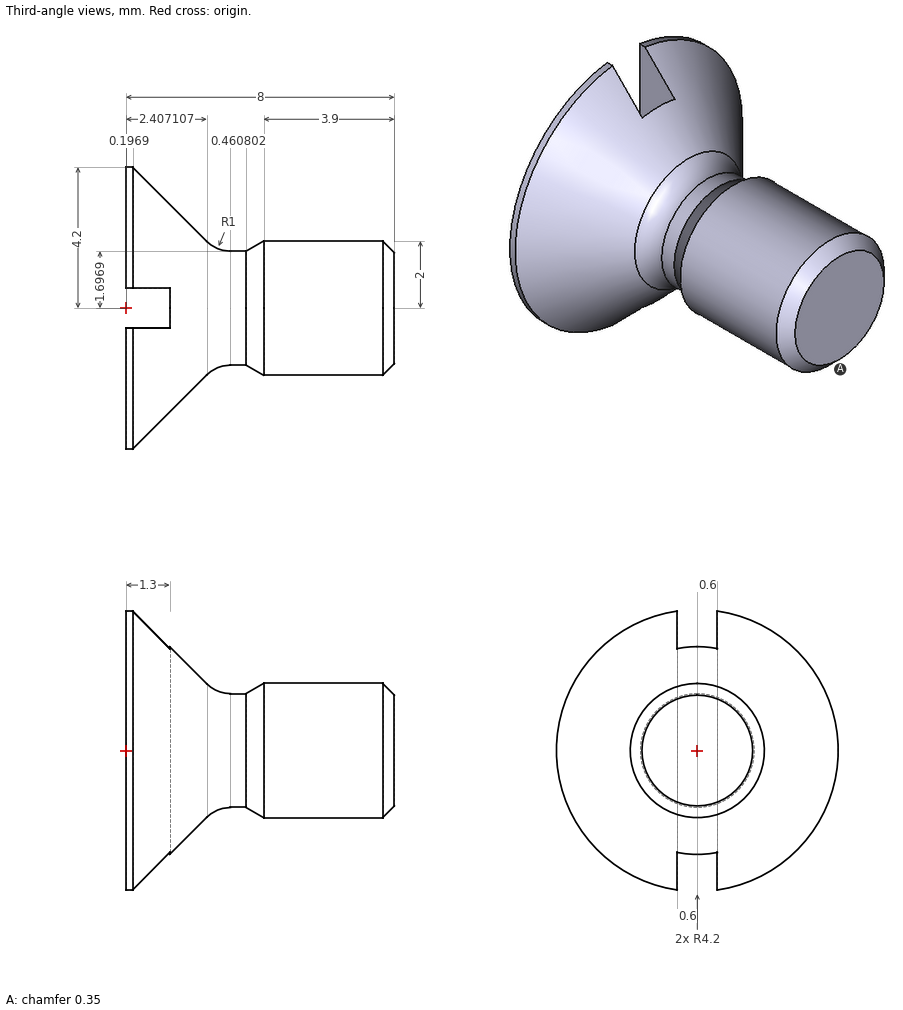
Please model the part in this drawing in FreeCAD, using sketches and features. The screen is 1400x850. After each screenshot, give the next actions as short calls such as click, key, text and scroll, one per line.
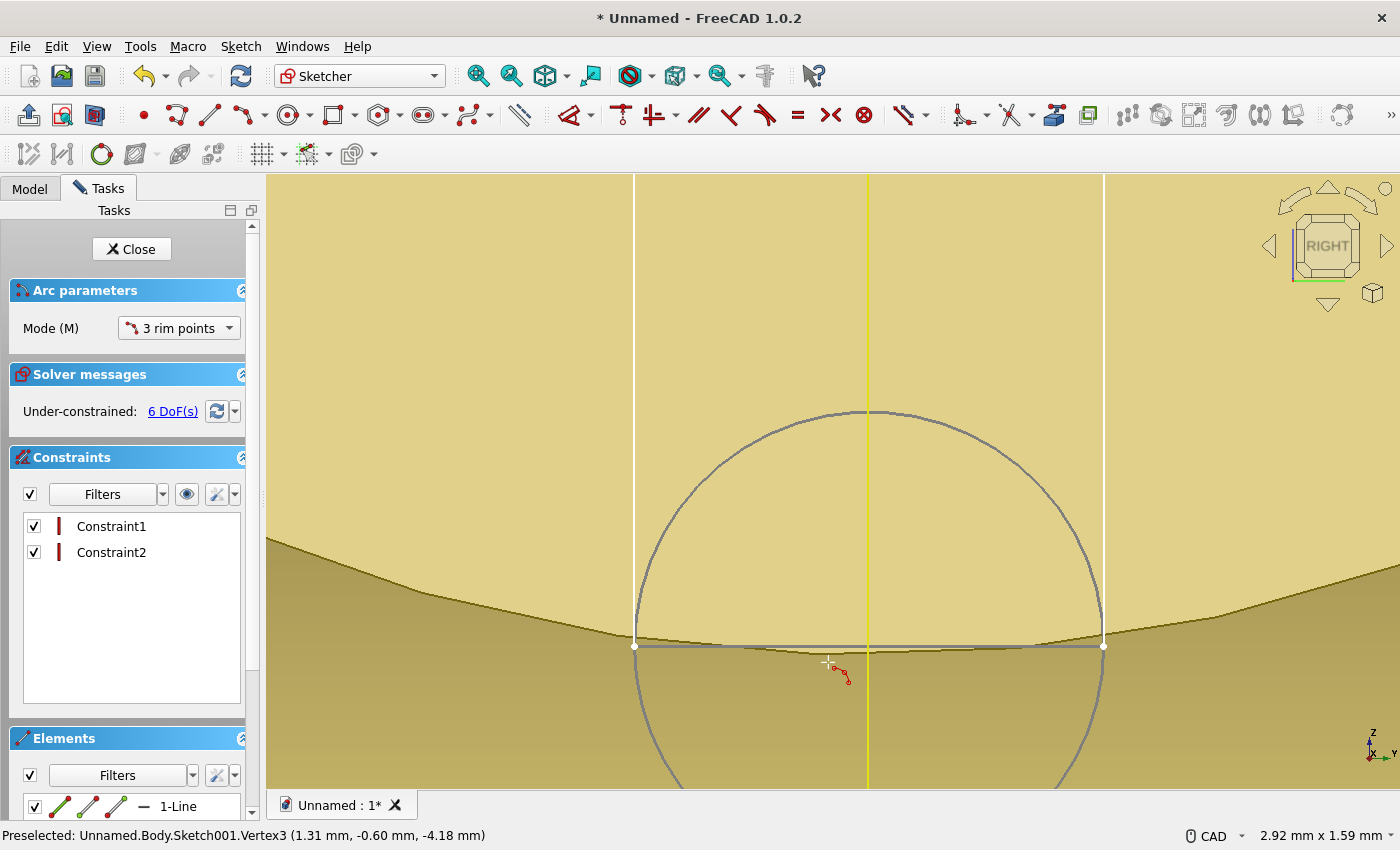
click(821, 654)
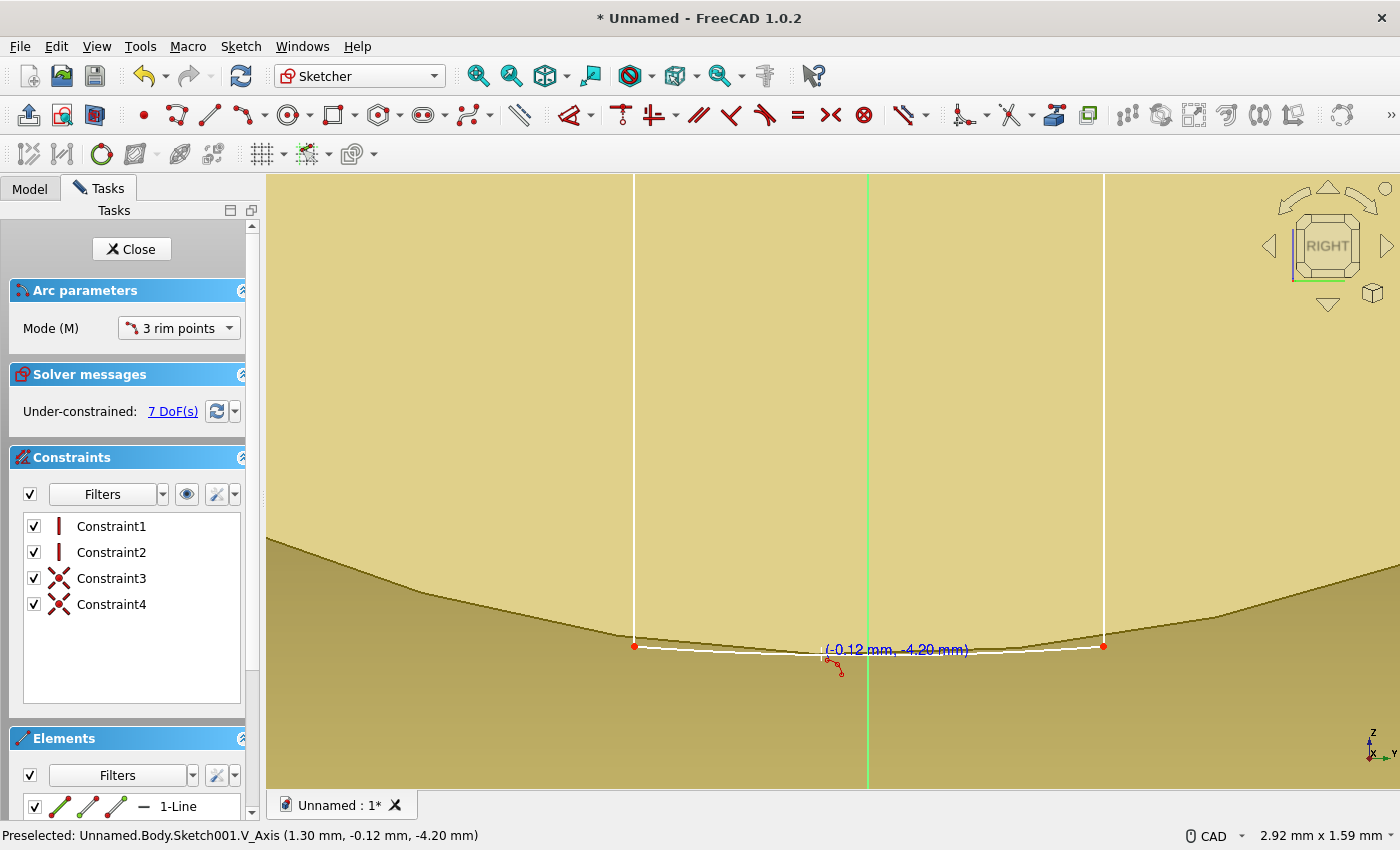
scroll(752, 663, down, 11)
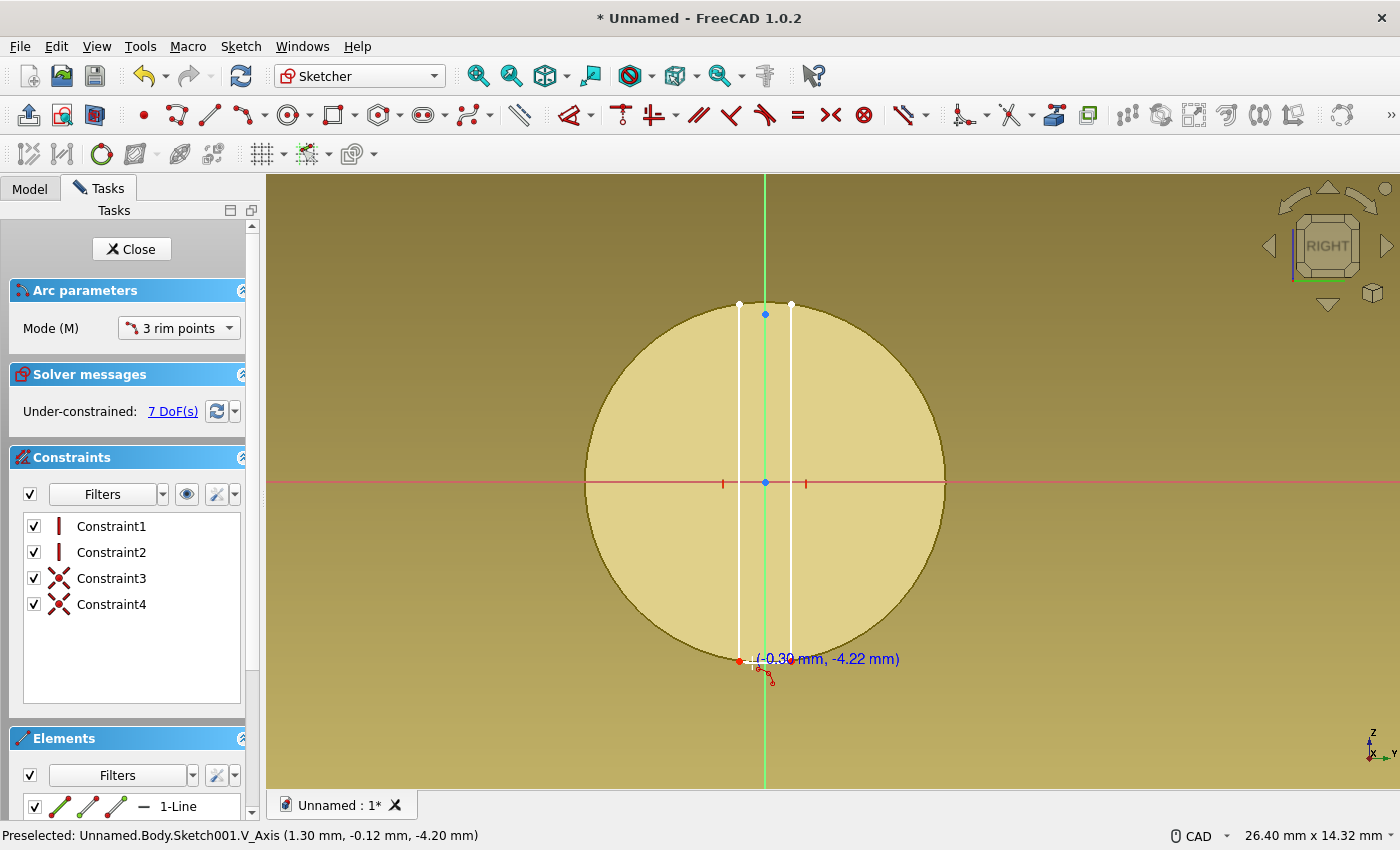
click(739, 305)
click(791, 305)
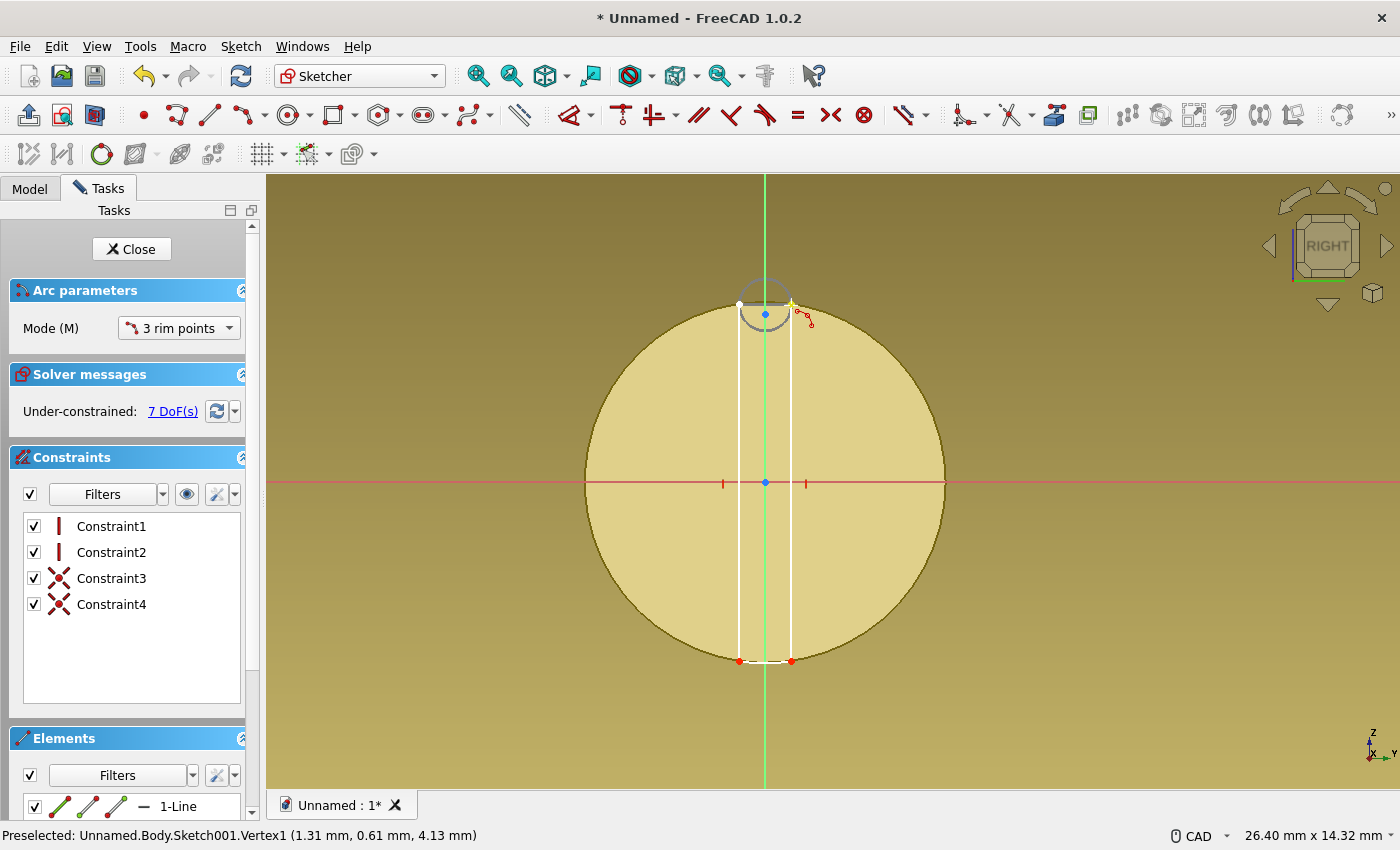
scroll(770, 302, up, 11)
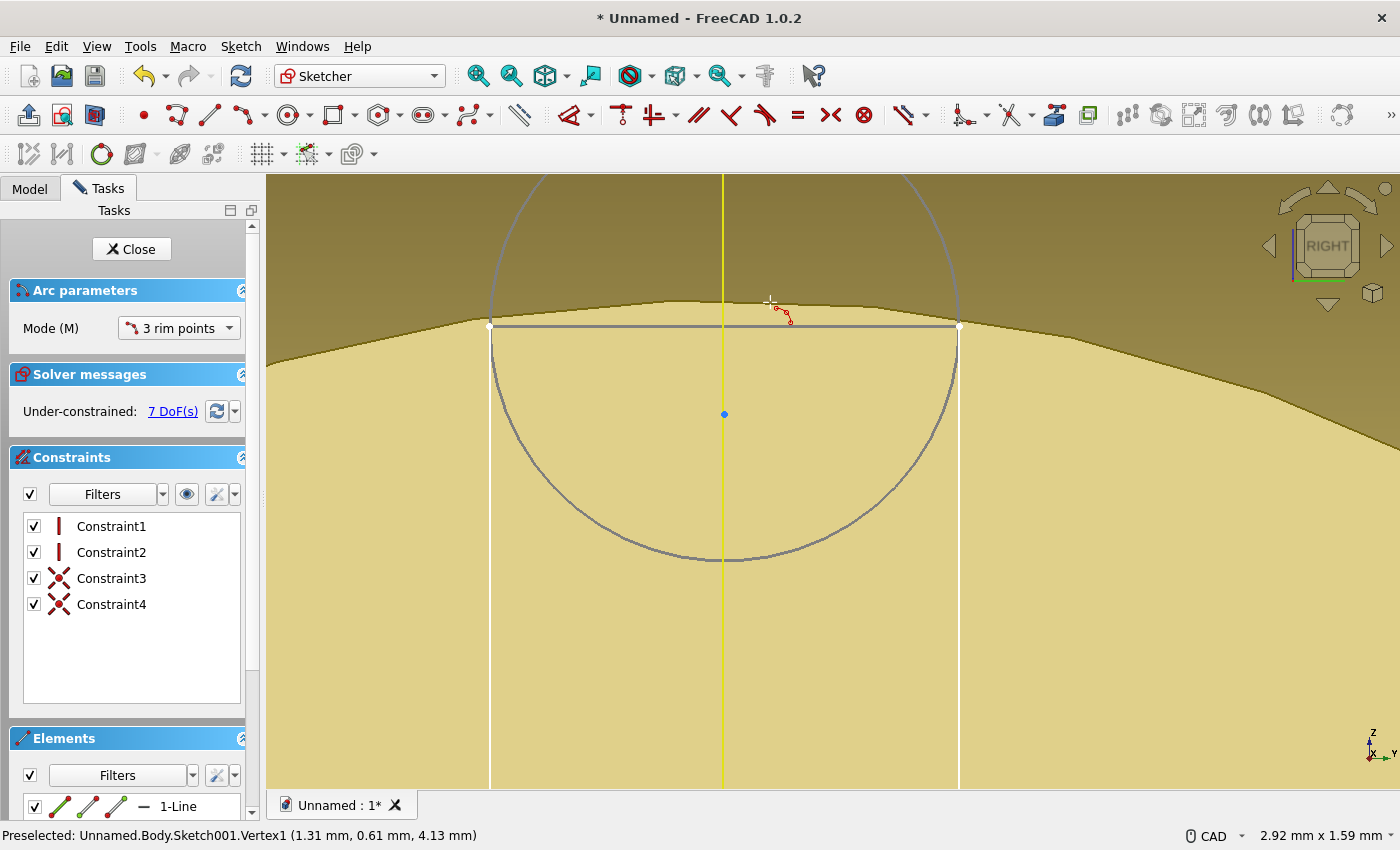
click(770, 301)
key(Escape)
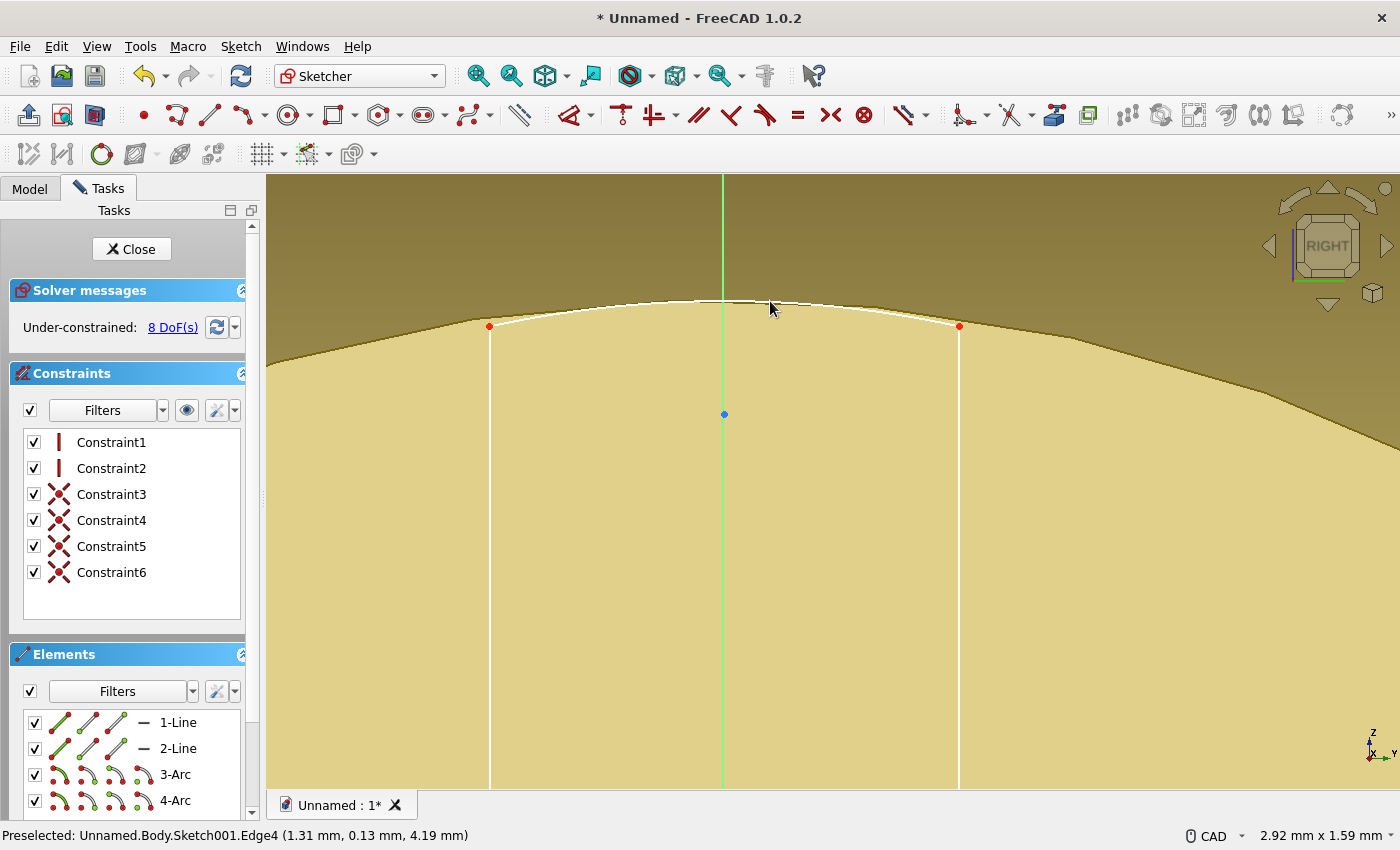
scroll(770, 301, down, 11)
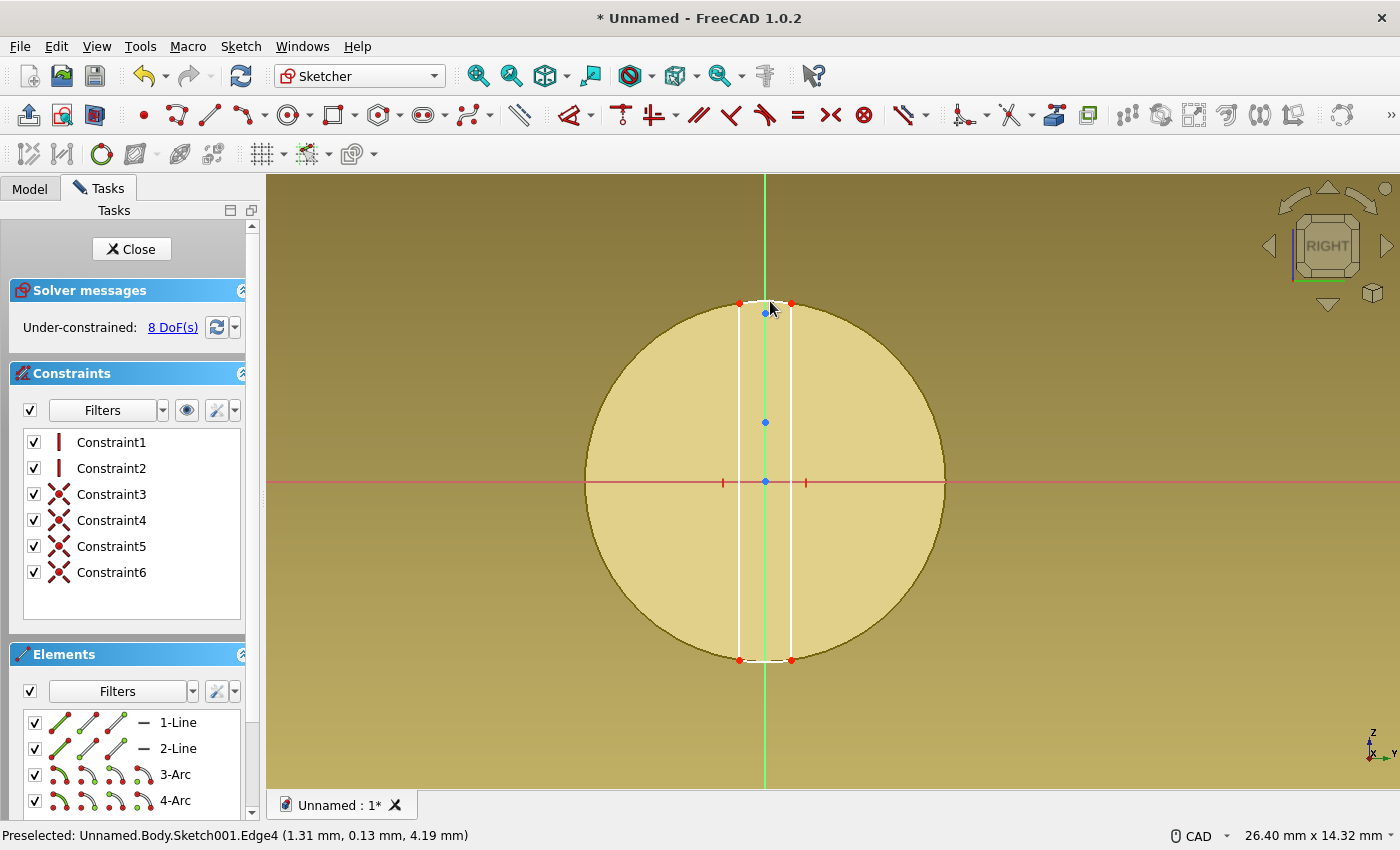
scroll(755, 662, up, 2)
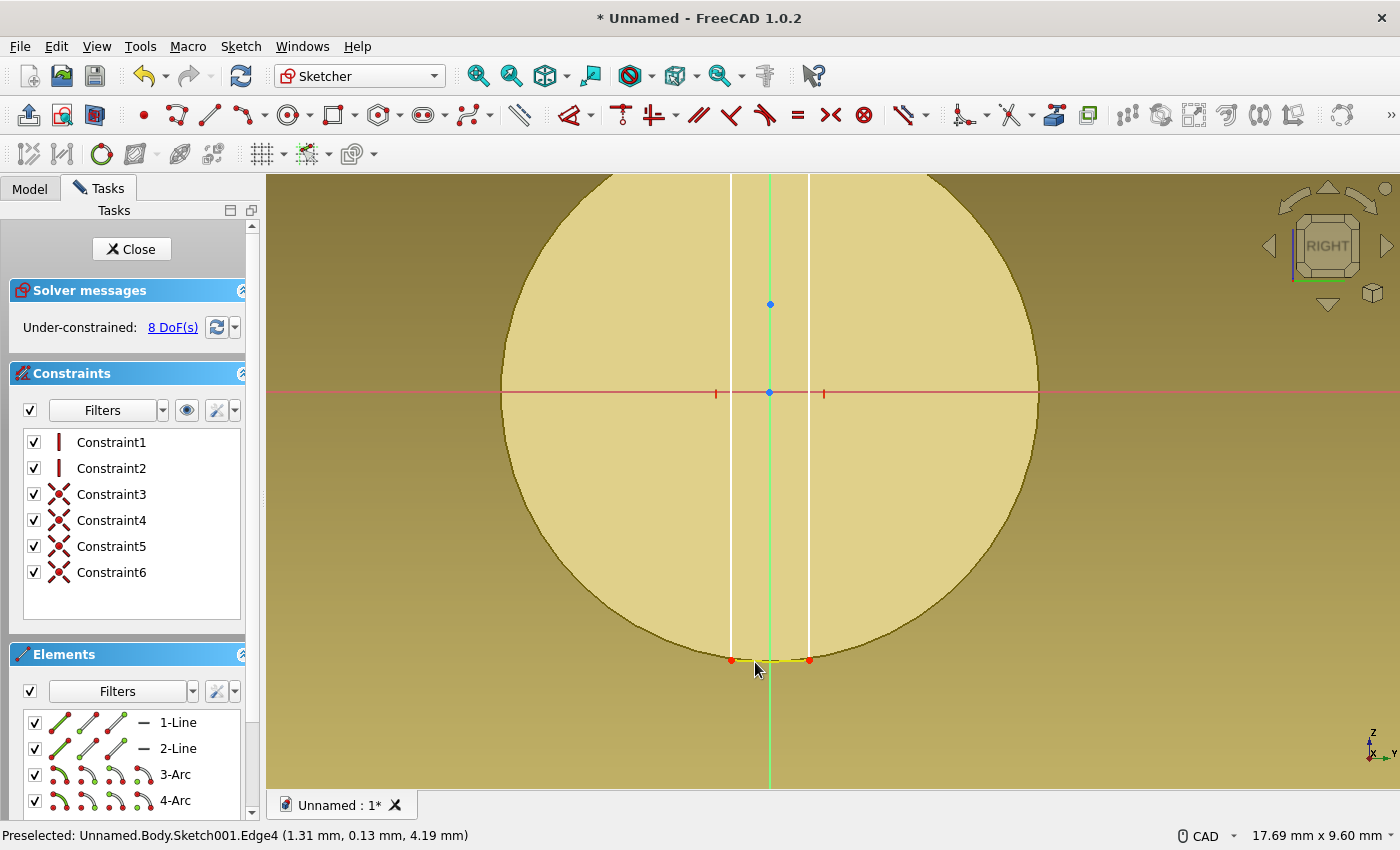
click(755, 661)